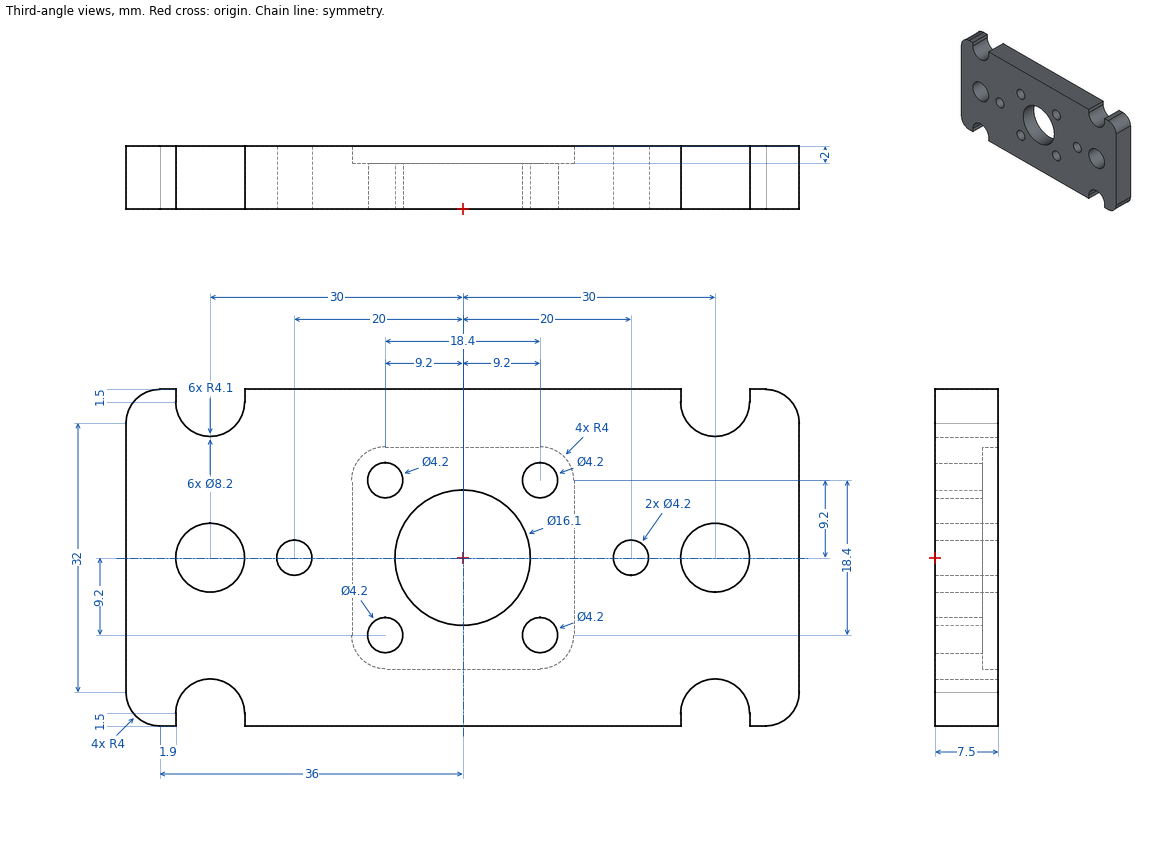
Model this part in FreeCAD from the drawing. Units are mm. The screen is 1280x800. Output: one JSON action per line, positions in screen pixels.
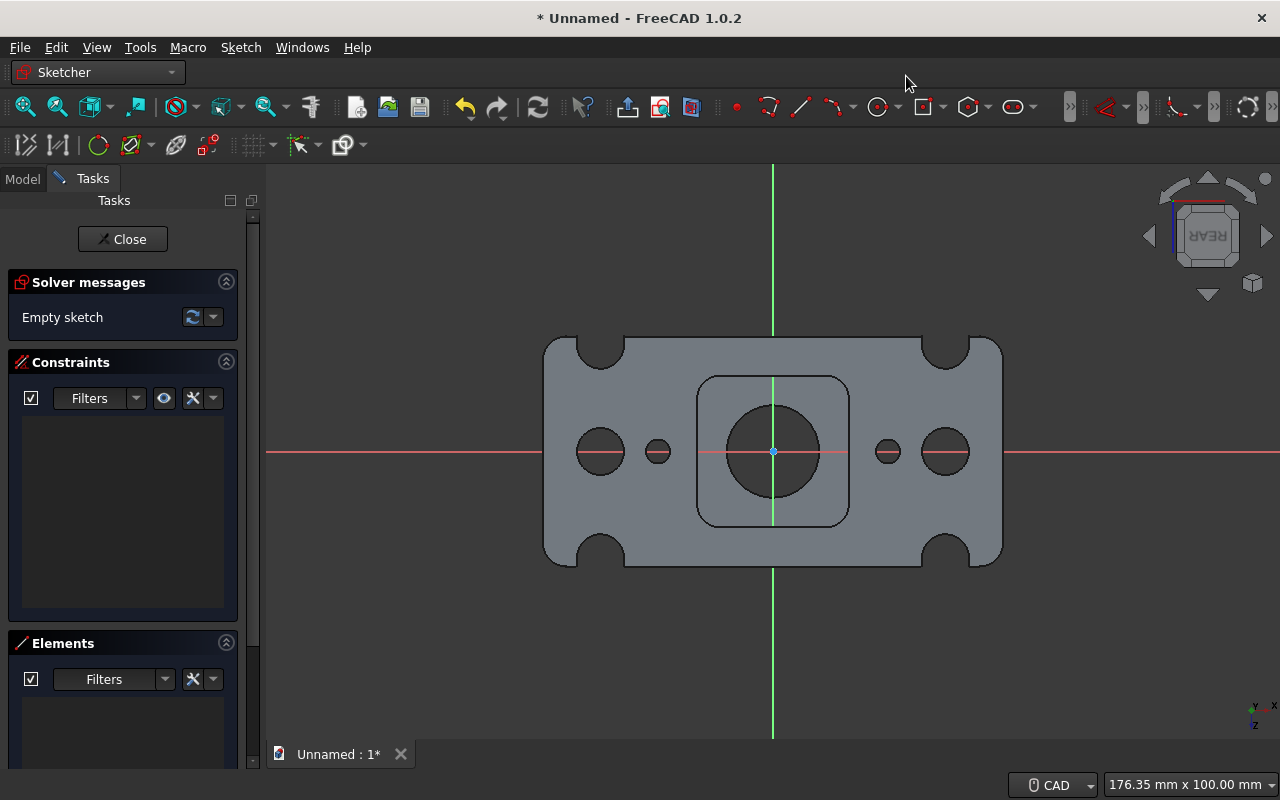
{"action": "left_click", "coordinate": [692, 108]}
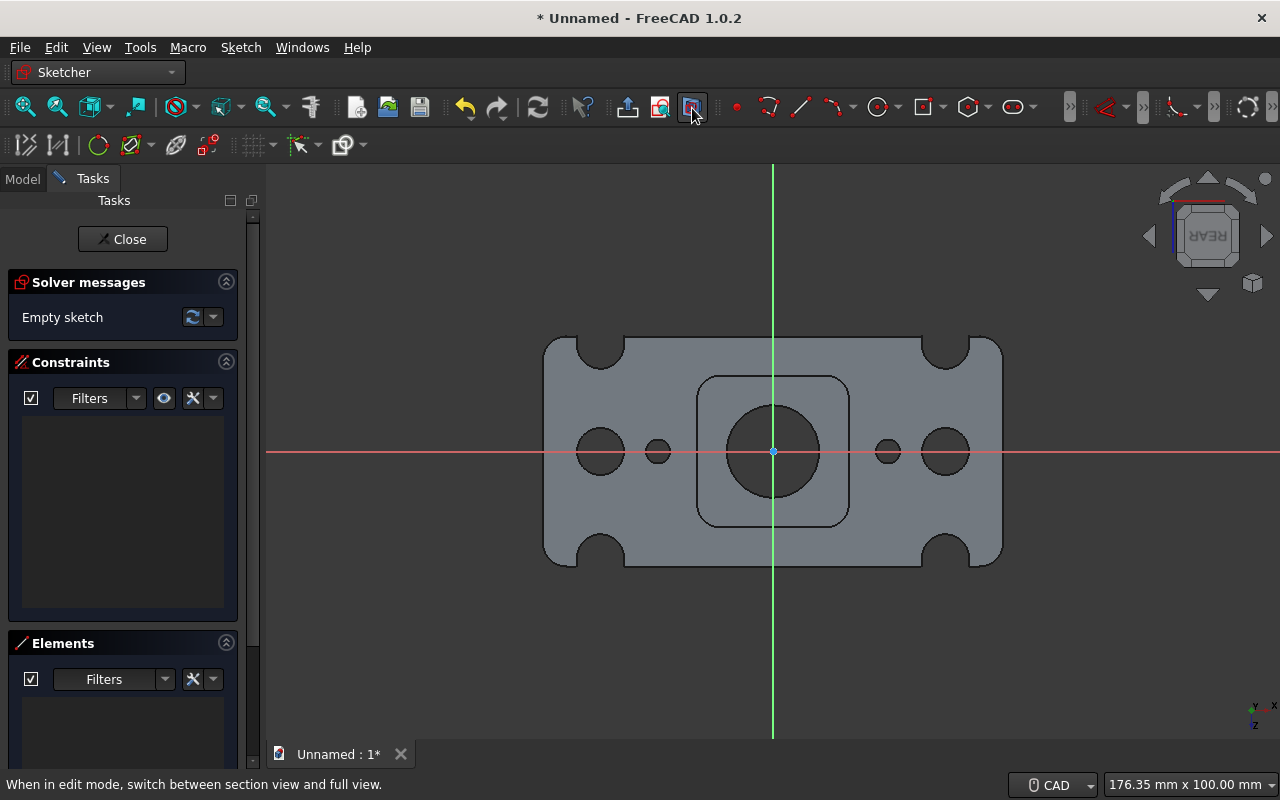
{"action": "scroll", "coordinate": [721, 395], "scroll_direction": "up", "scroll_amount": 14}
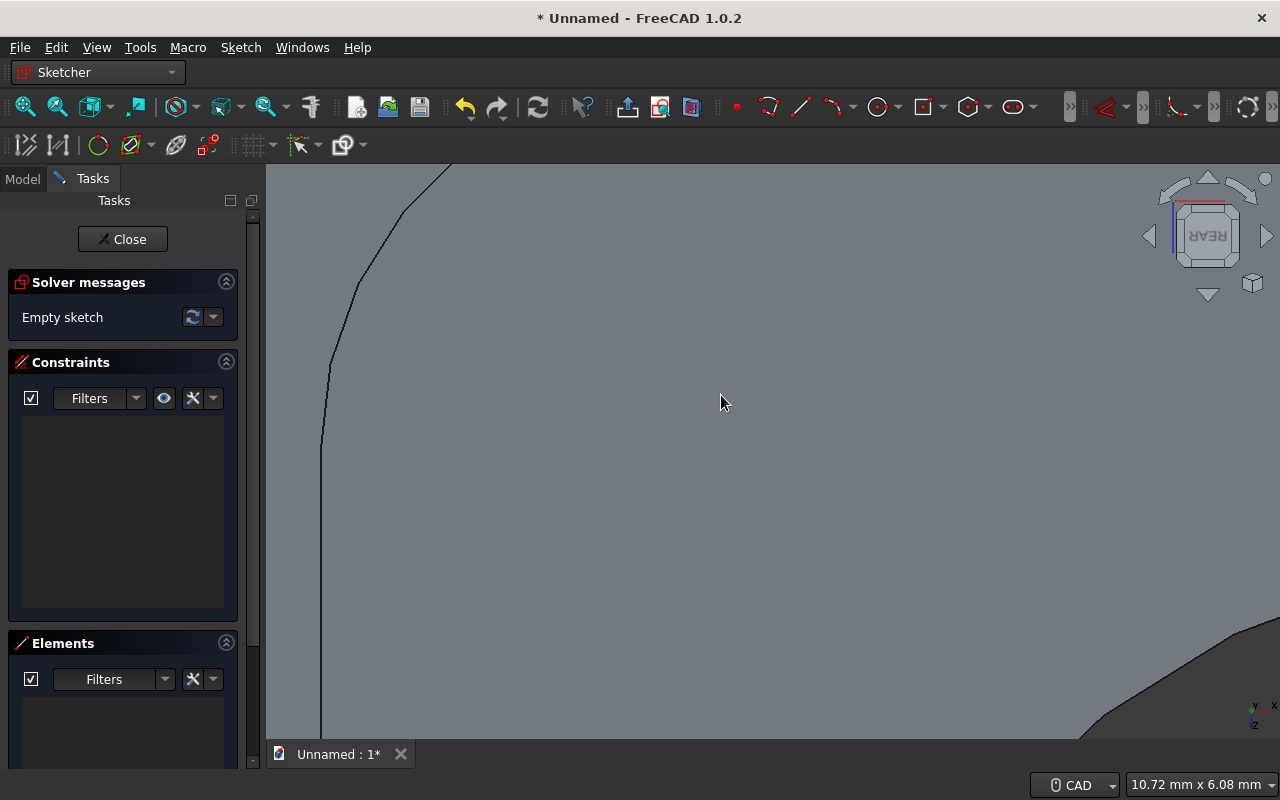
{"action": "left_click", "coordinate": [878, 108]}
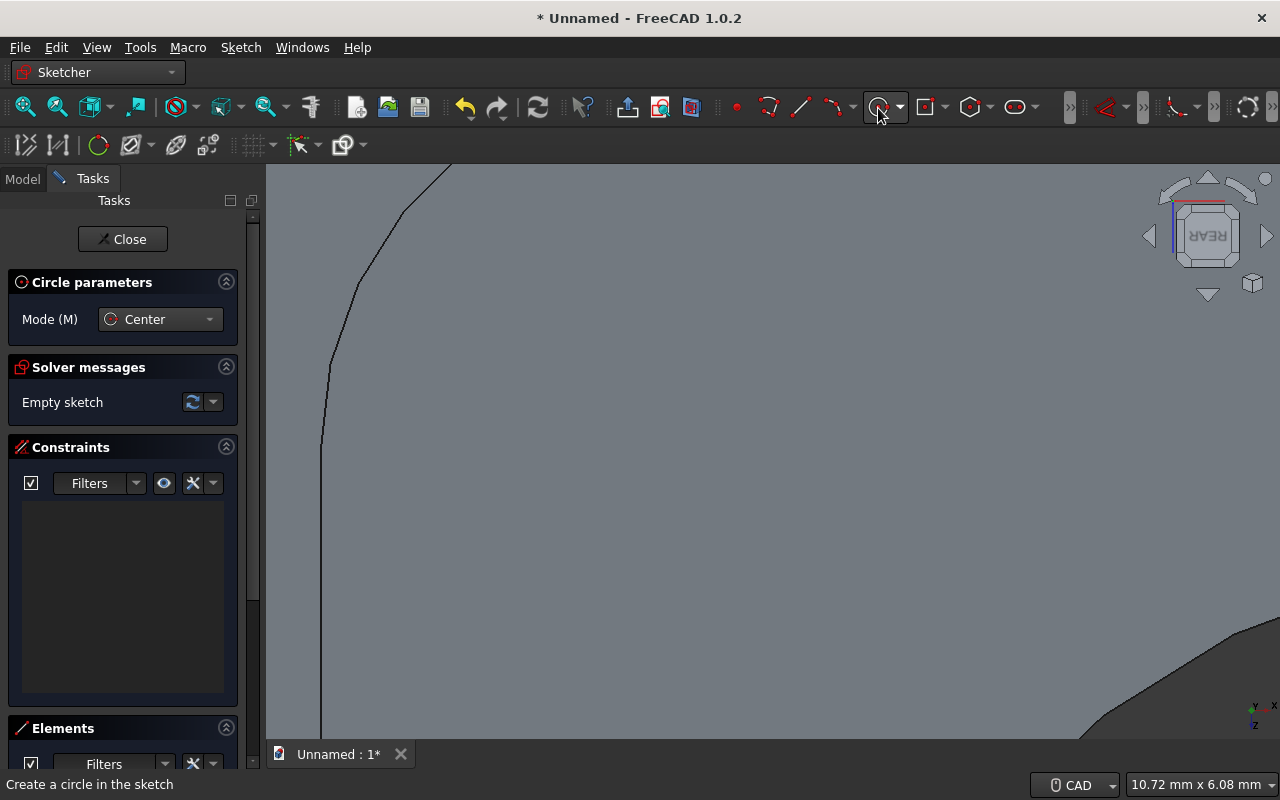
{"action": "left_click", "coordinate": [699, 448]}
{"action": "mouse_move", "coordinate": [840, 308]}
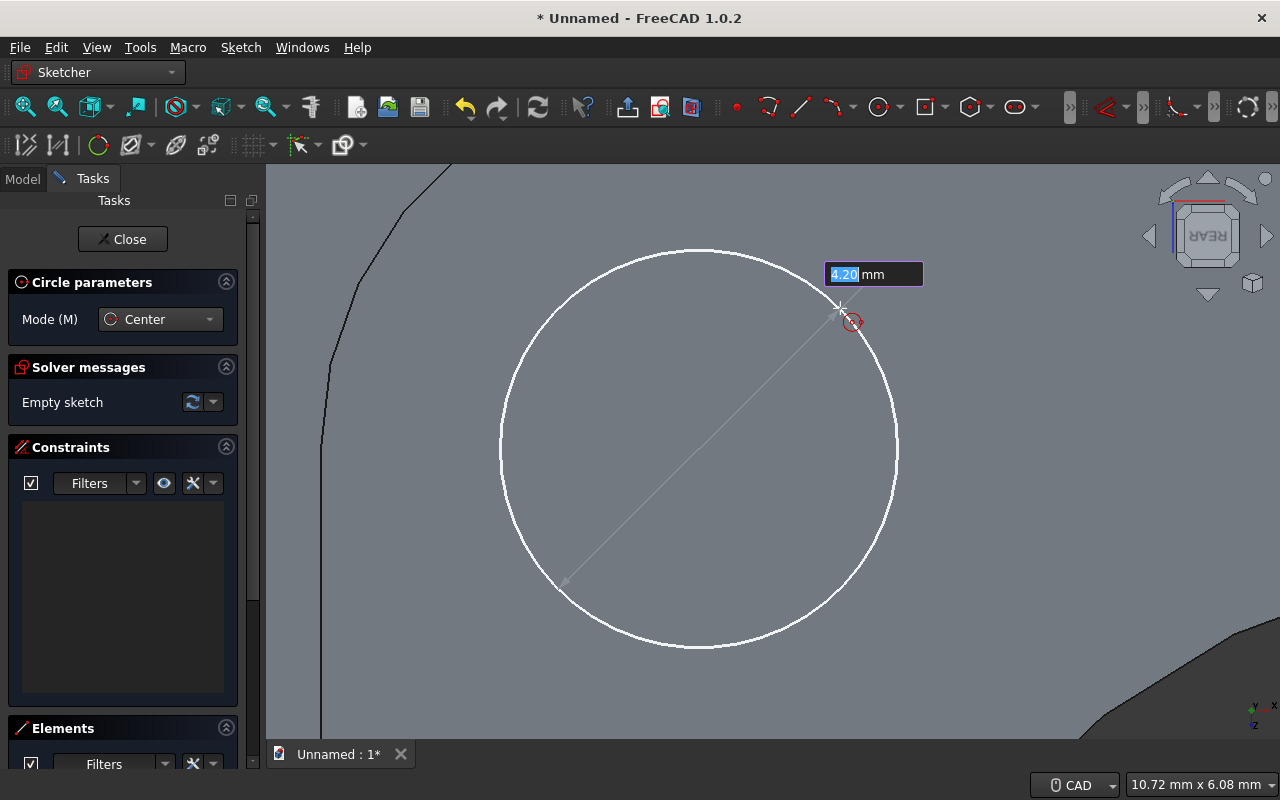
{"action": "type", "text": "4.2"}
{"action": "key", "text": "Return"}
{"action": "key", "text": "Escape"}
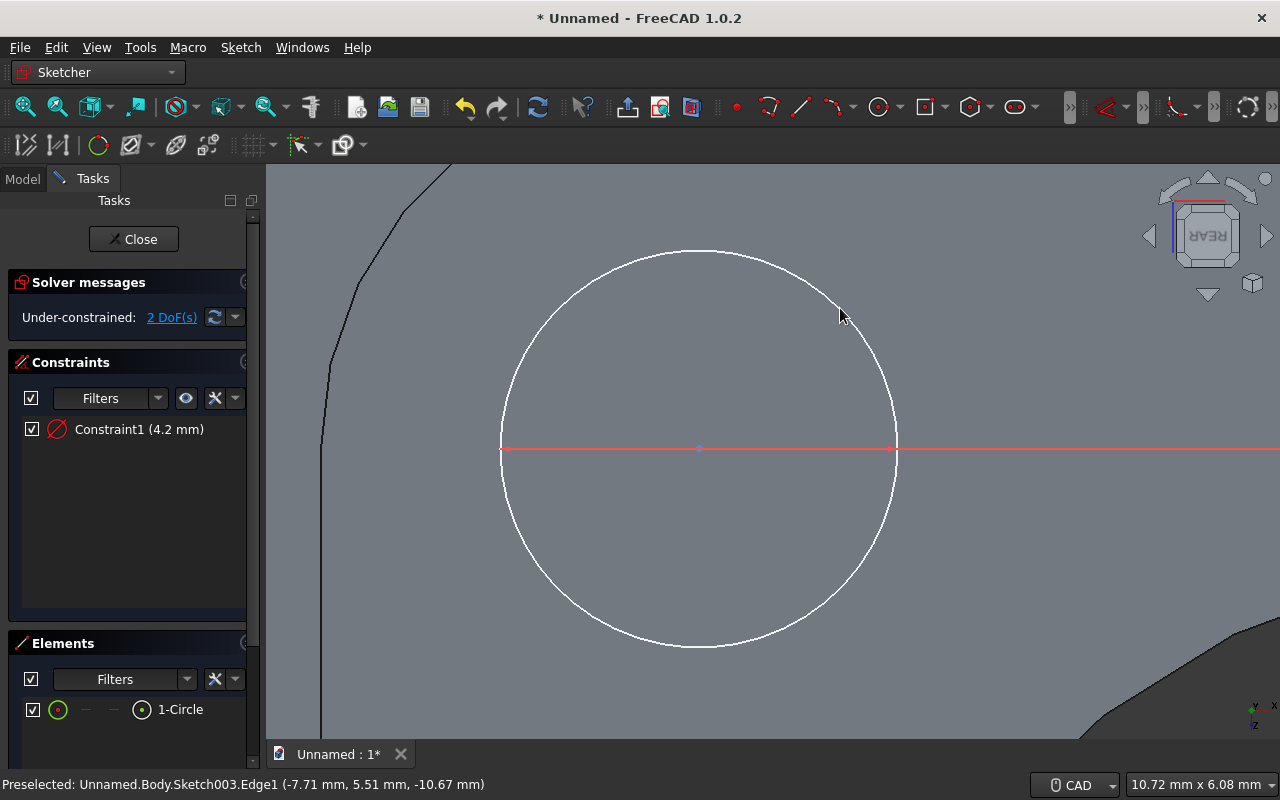
{"action": "left_click", "coordinate": [1106, 108]}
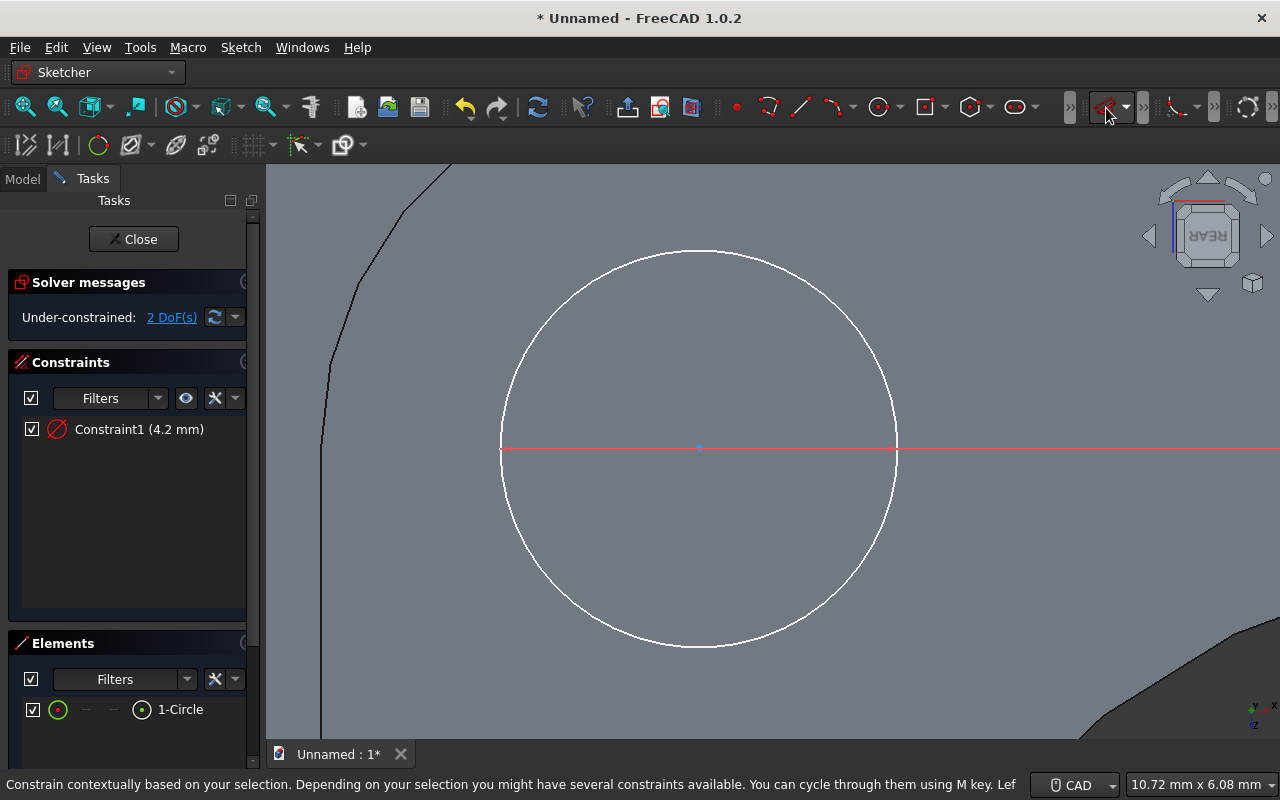
{"action": "left_click", "coordinate": [699, 449]}
{"action": "left_click", "coordinate": [811, 415]}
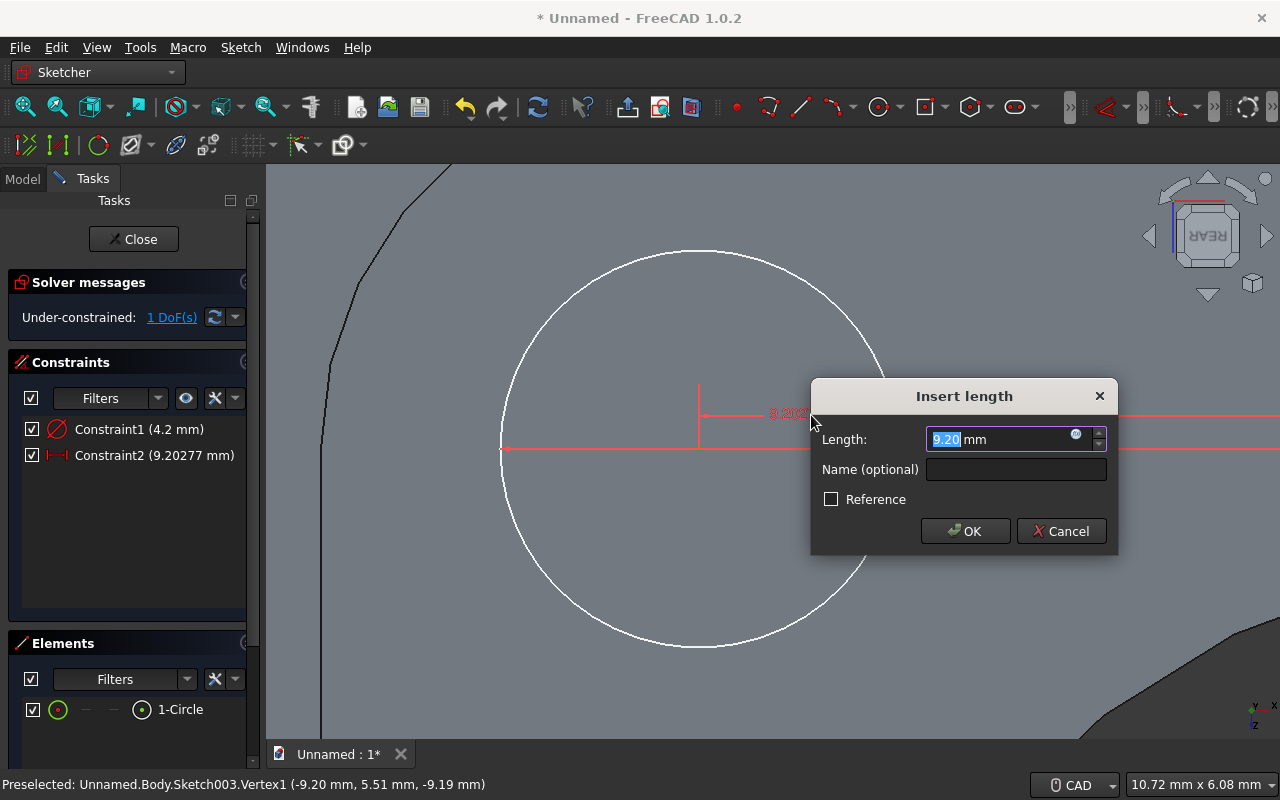
{"action": "type", "text": "9.2"}
{"action": "key", "text": "Return"}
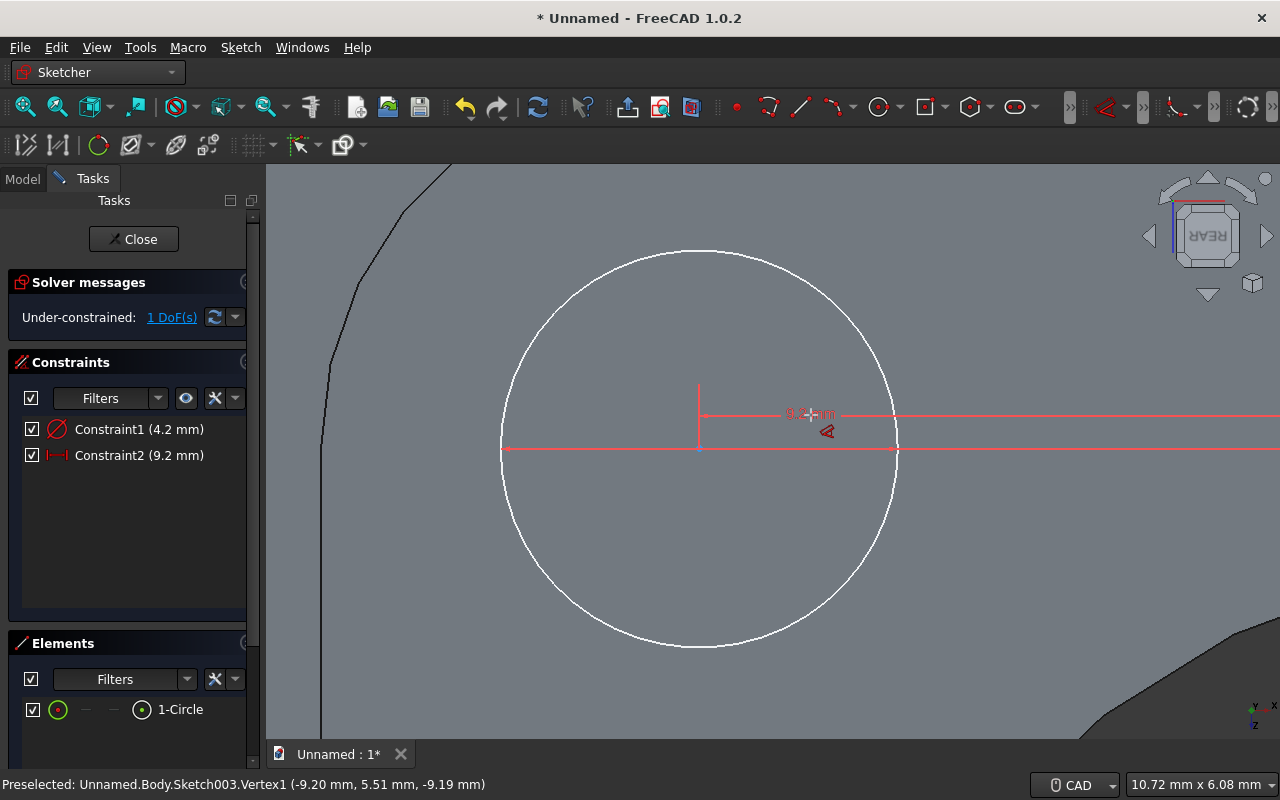
{"action": "left_click", "coordinate": [699, 449]}
{"action": "left_click", "coordinate": [665, 580]}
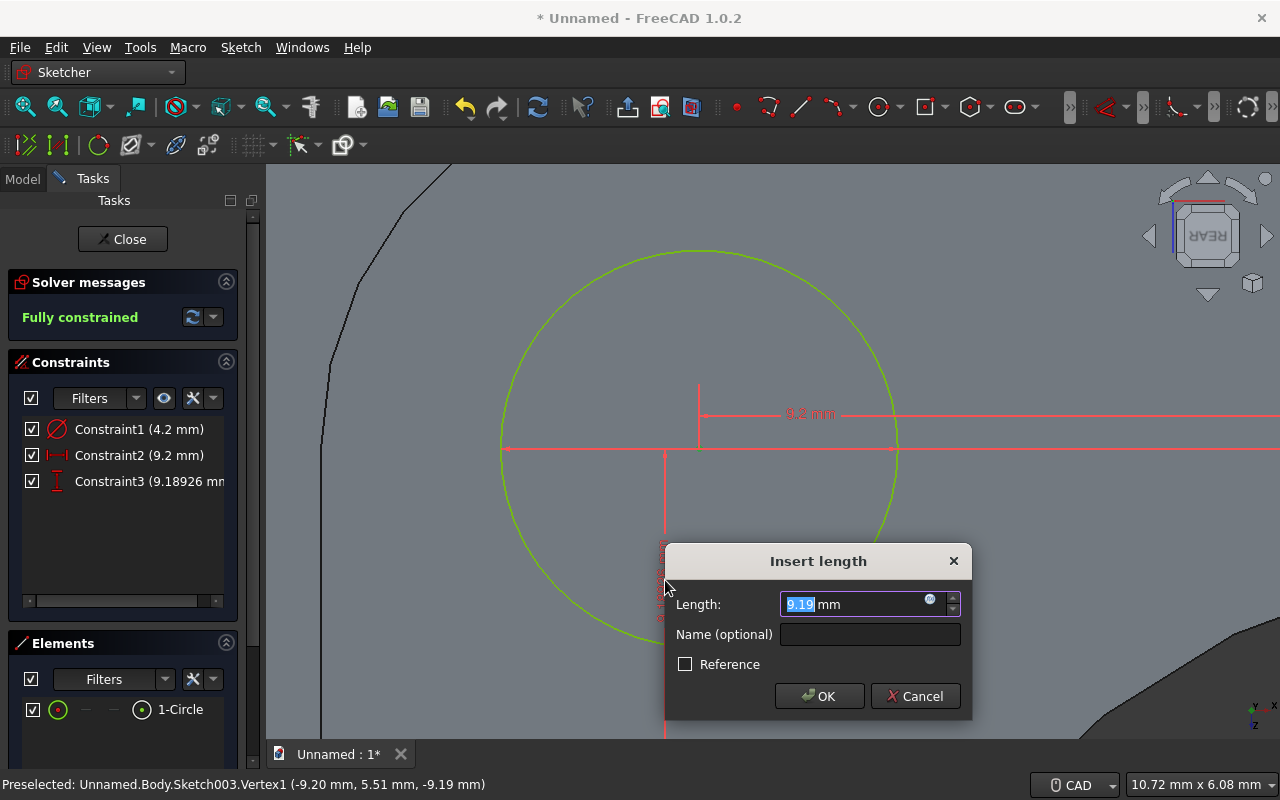
{"action": "type", "text": "9.2"}
{"action": "key", "text": "Return"}
{"action": "key", "text": "Escape"}